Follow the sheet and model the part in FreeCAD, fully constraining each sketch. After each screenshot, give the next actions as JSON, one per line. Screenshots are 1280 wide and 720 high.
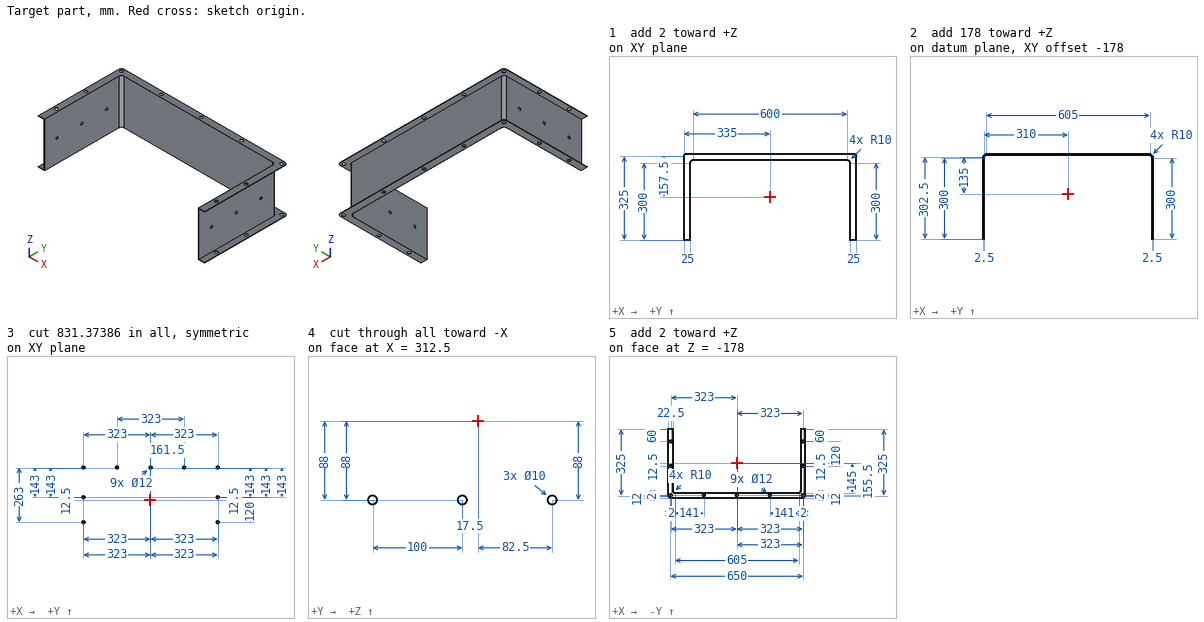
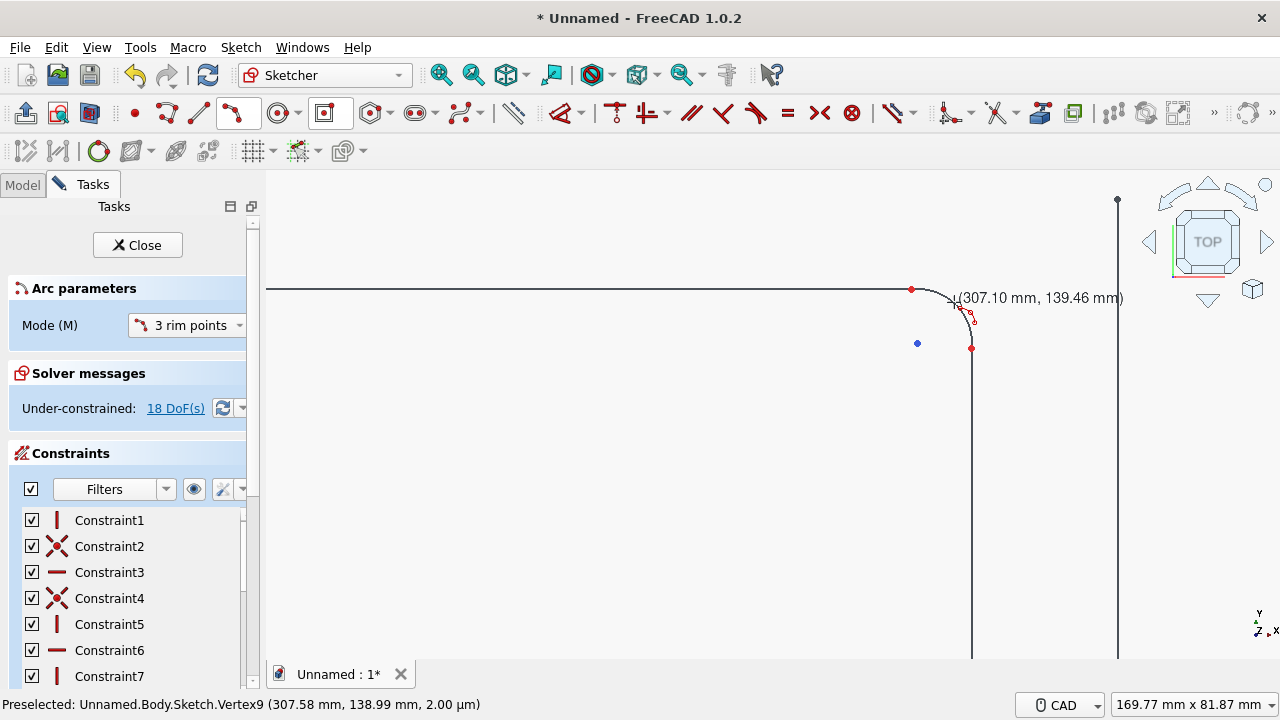
{"action": "scroll", "coordinate": [953, 302], "scroll_direction": "down", "scroll_amount": 10}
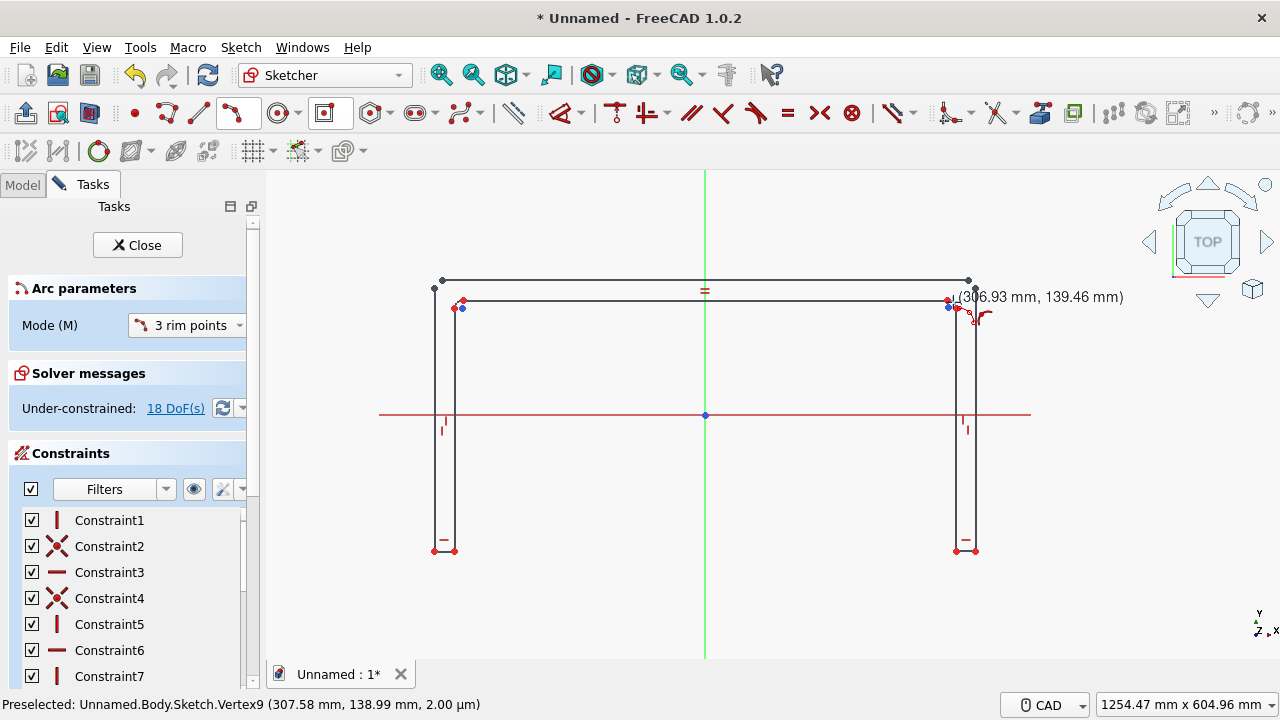
{"action": "scroll", "coordinate": [976, 288], "scroll_direction": "up", "scroll_amount": 2}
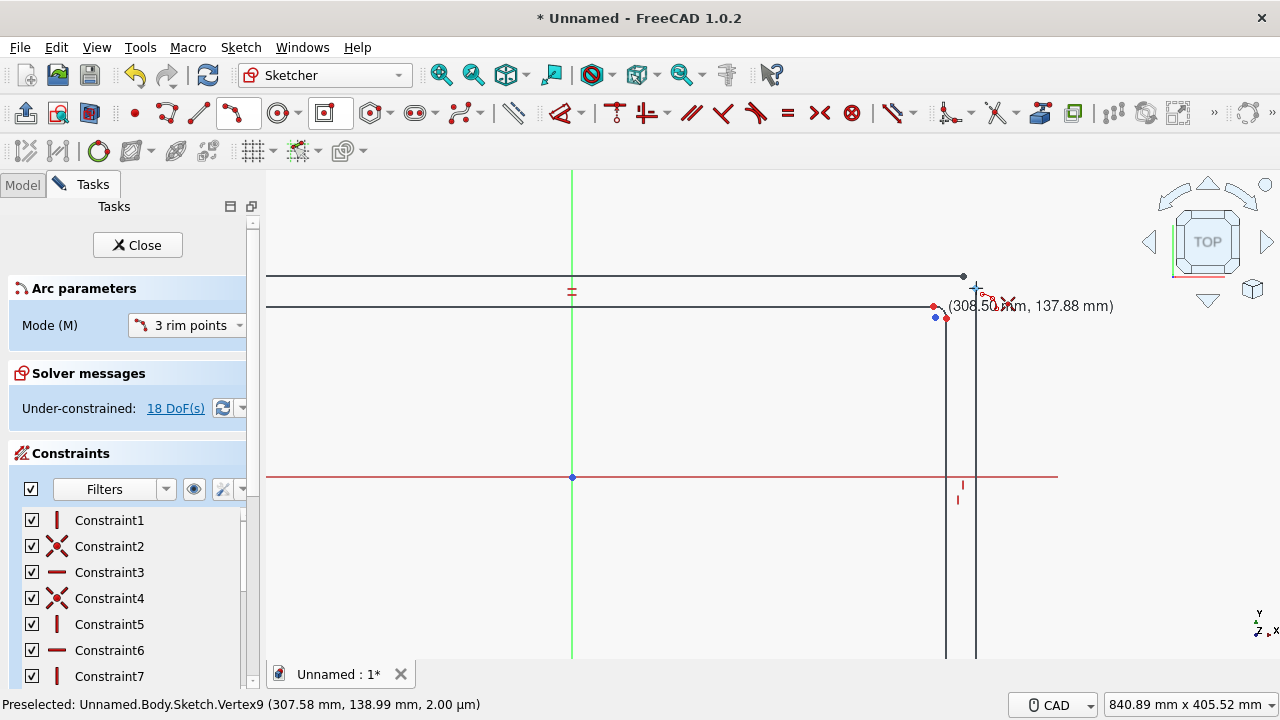
{"action": "left_click", "coordinate": [976, 289]}
{"action": "left_click", "coordinate": [964, 276]}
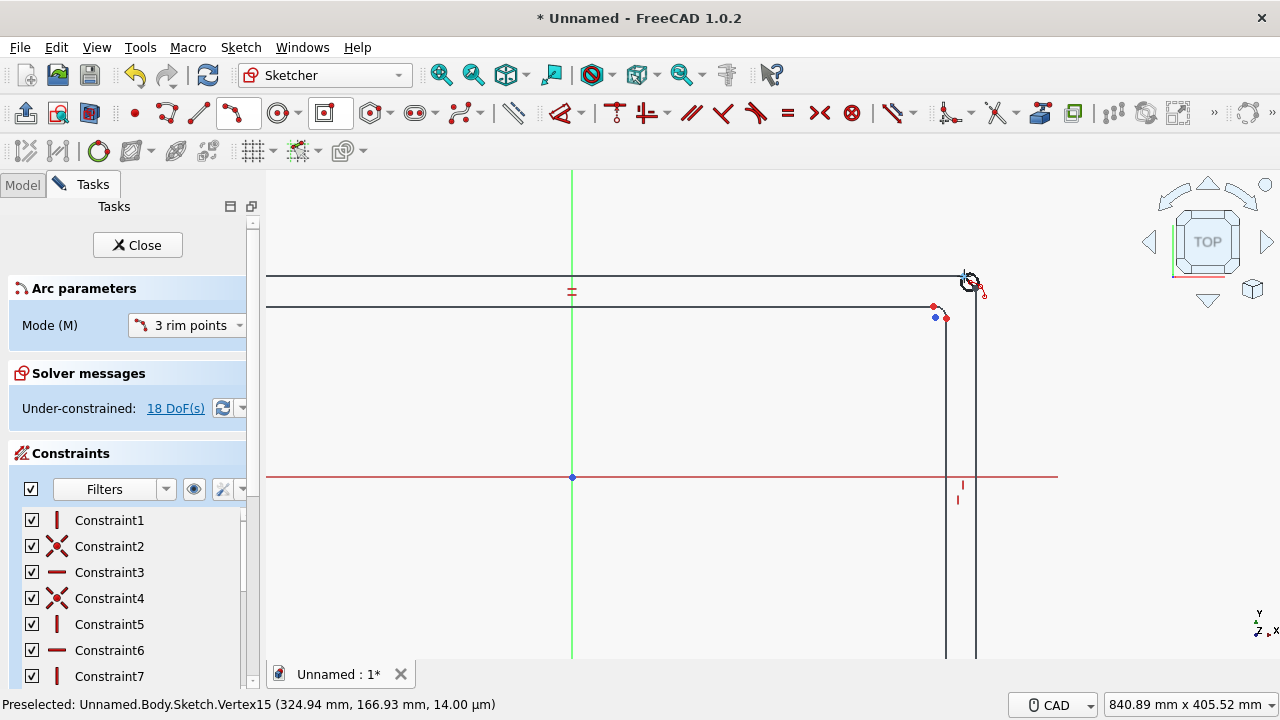
{"action": "scroll", "coordinate": [973, 279], "scroll_direction": "up", "scroll_amount": 8}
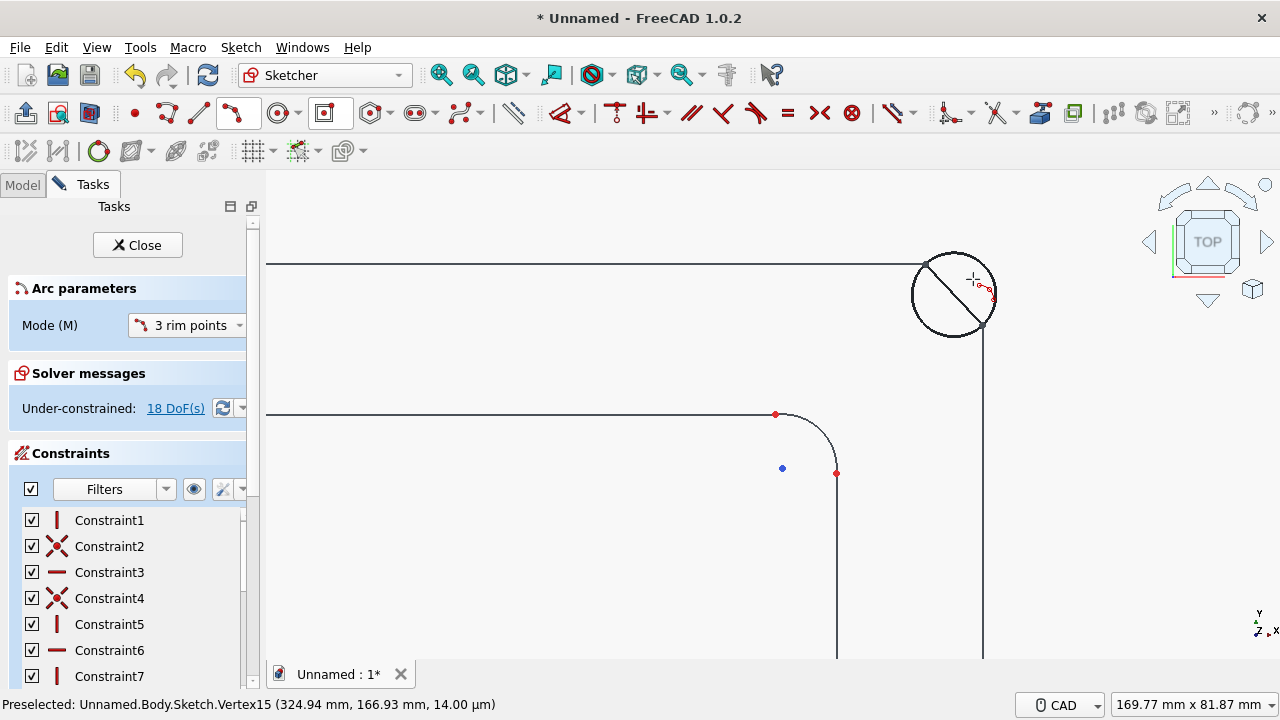
{"action": "left_click", "coordinate": [968, 278]}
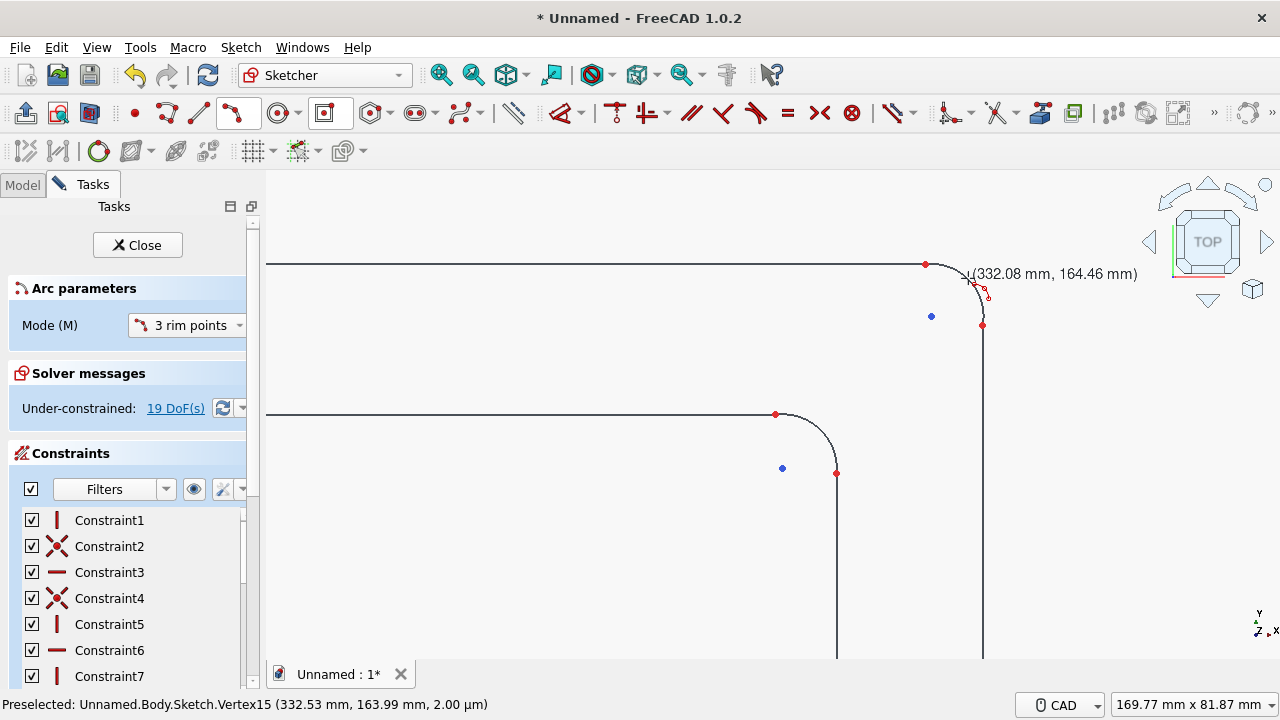
{"action": "scroll", "coordinate": [974, 282], "scroll_direction": "down", "scroll_amount": 10}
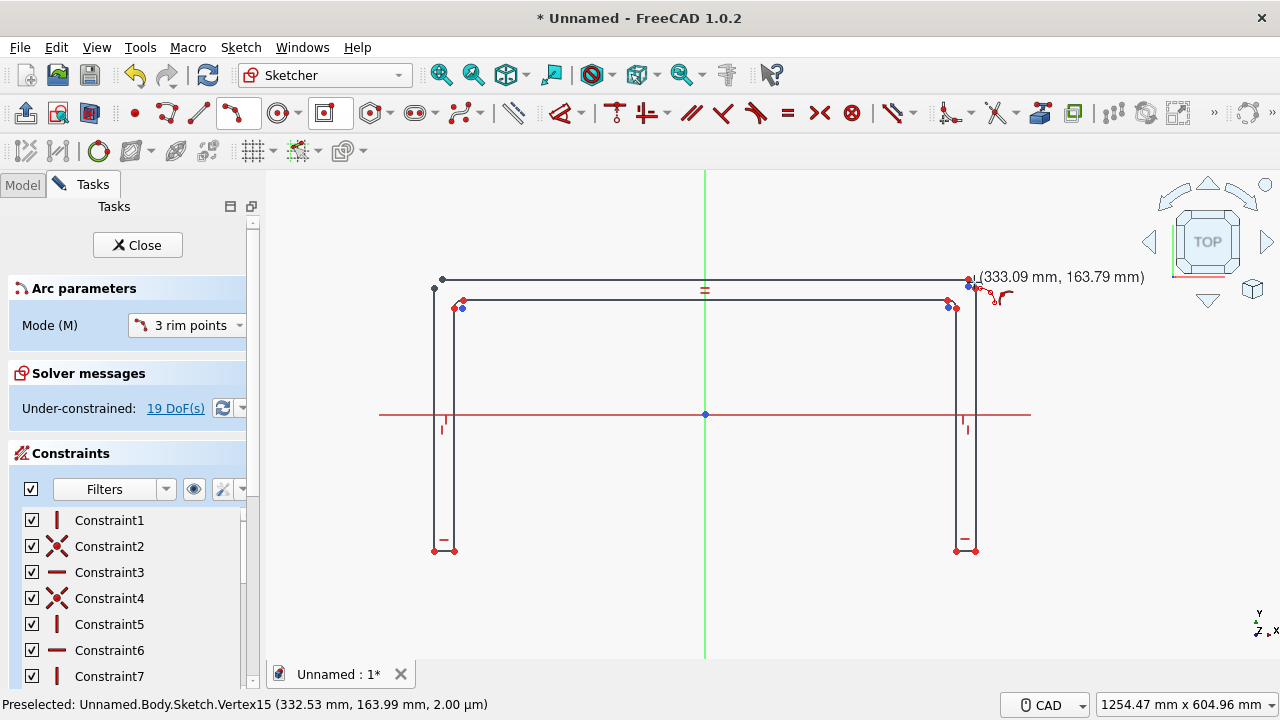
{"action": "scroll", "coordinate": [443, 279], "scroll_direction": "up", "scroll_amount": 2}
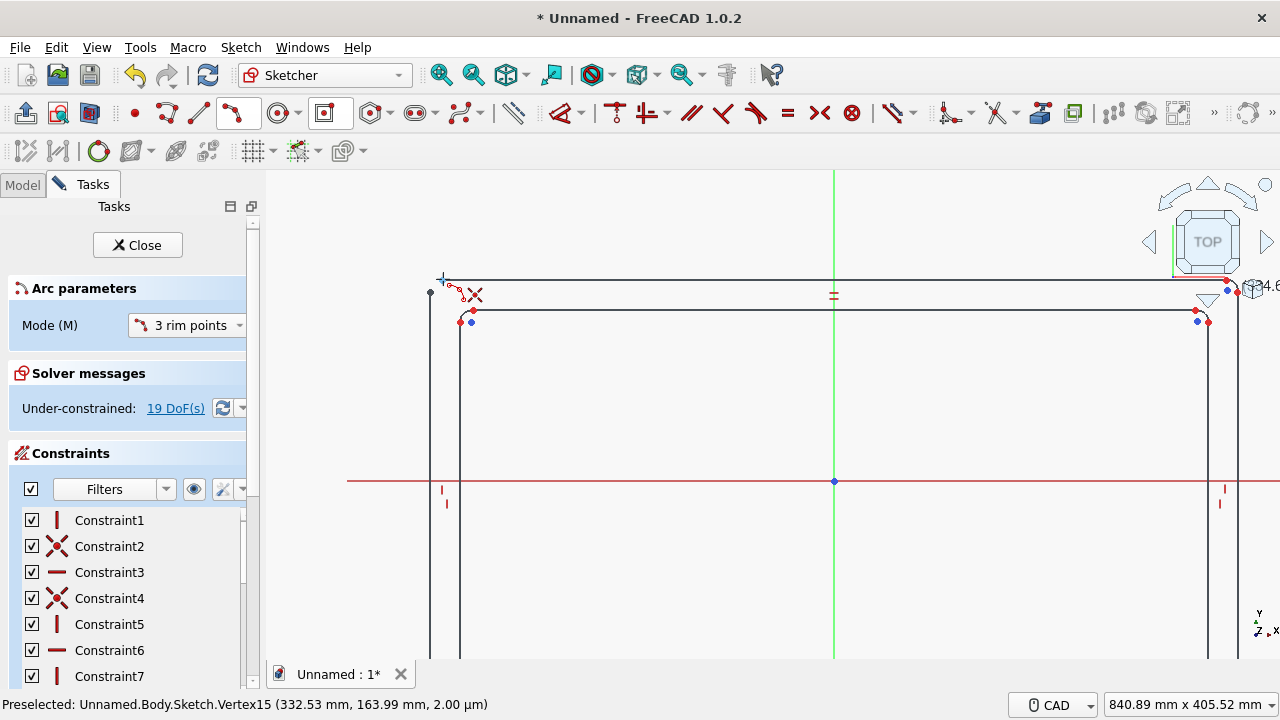
{"action": "left_click", "coordinate": [443, 280]}
{"action": "left_click", "coordinate": [430, 293]}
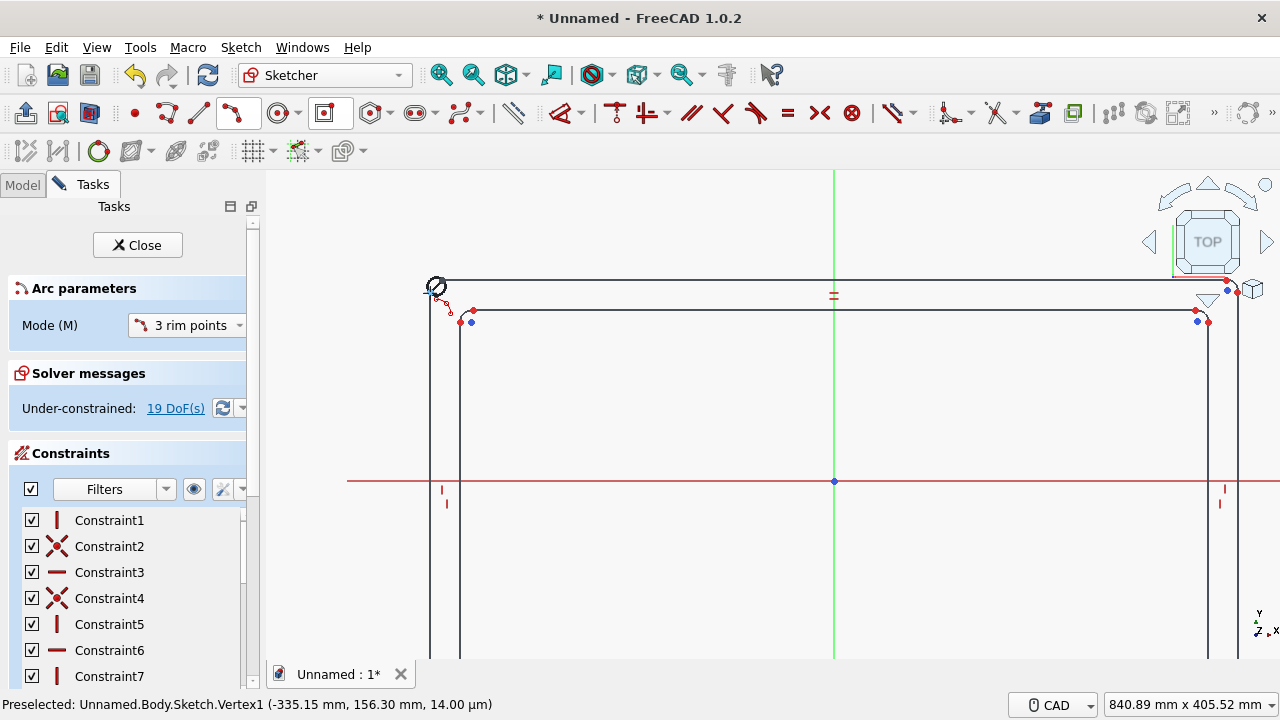
{"action": "scroll", "coordinate": [434, 283], "scroll_direction": "up", "scroll_amount": 8}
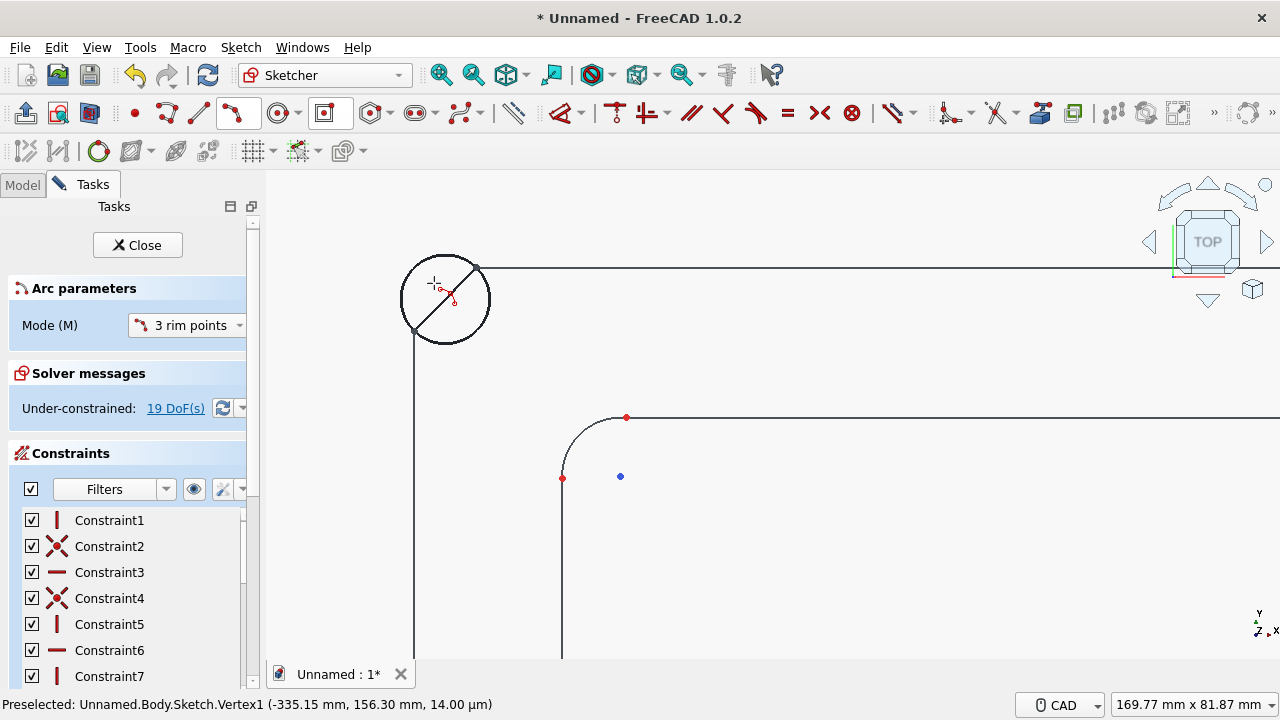
{"action": "left_click", "coordinate": [433, 282]}
{"action": "key", "text": "Escape"}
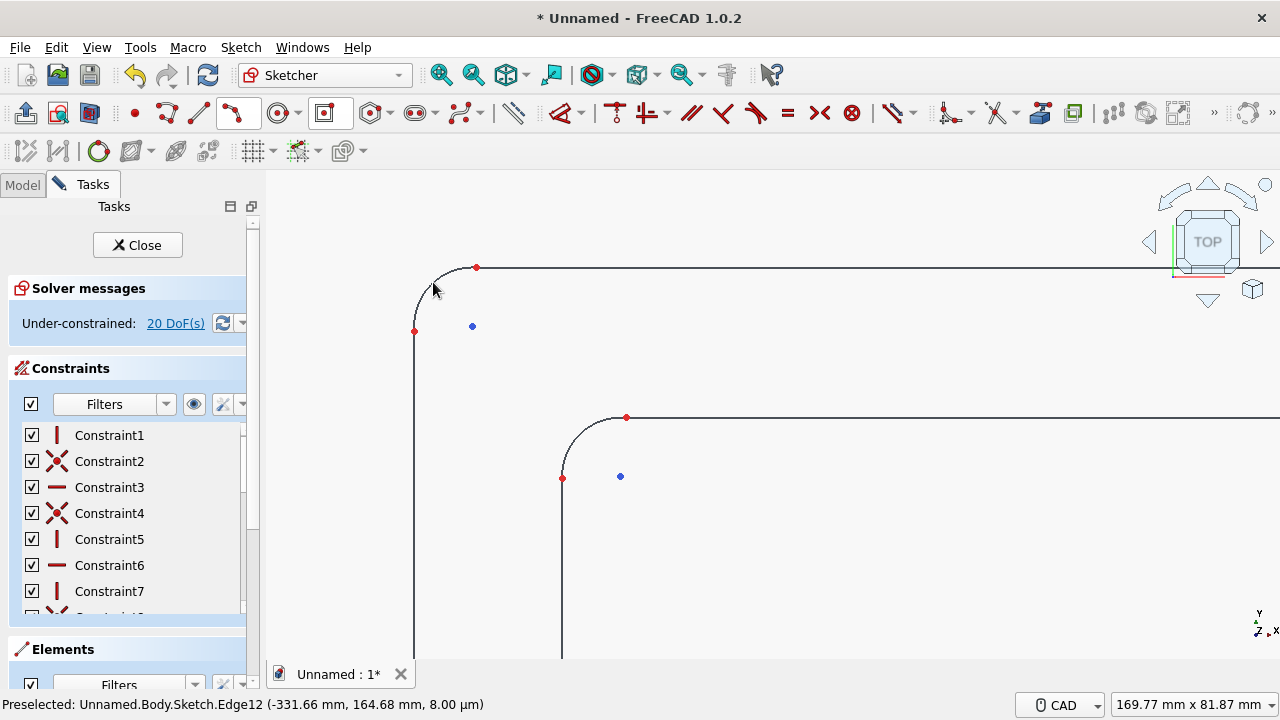
{"action": "scroll", "coordinate": [437, 281], "scroll_direction": "down", "scroll_amount": 10}